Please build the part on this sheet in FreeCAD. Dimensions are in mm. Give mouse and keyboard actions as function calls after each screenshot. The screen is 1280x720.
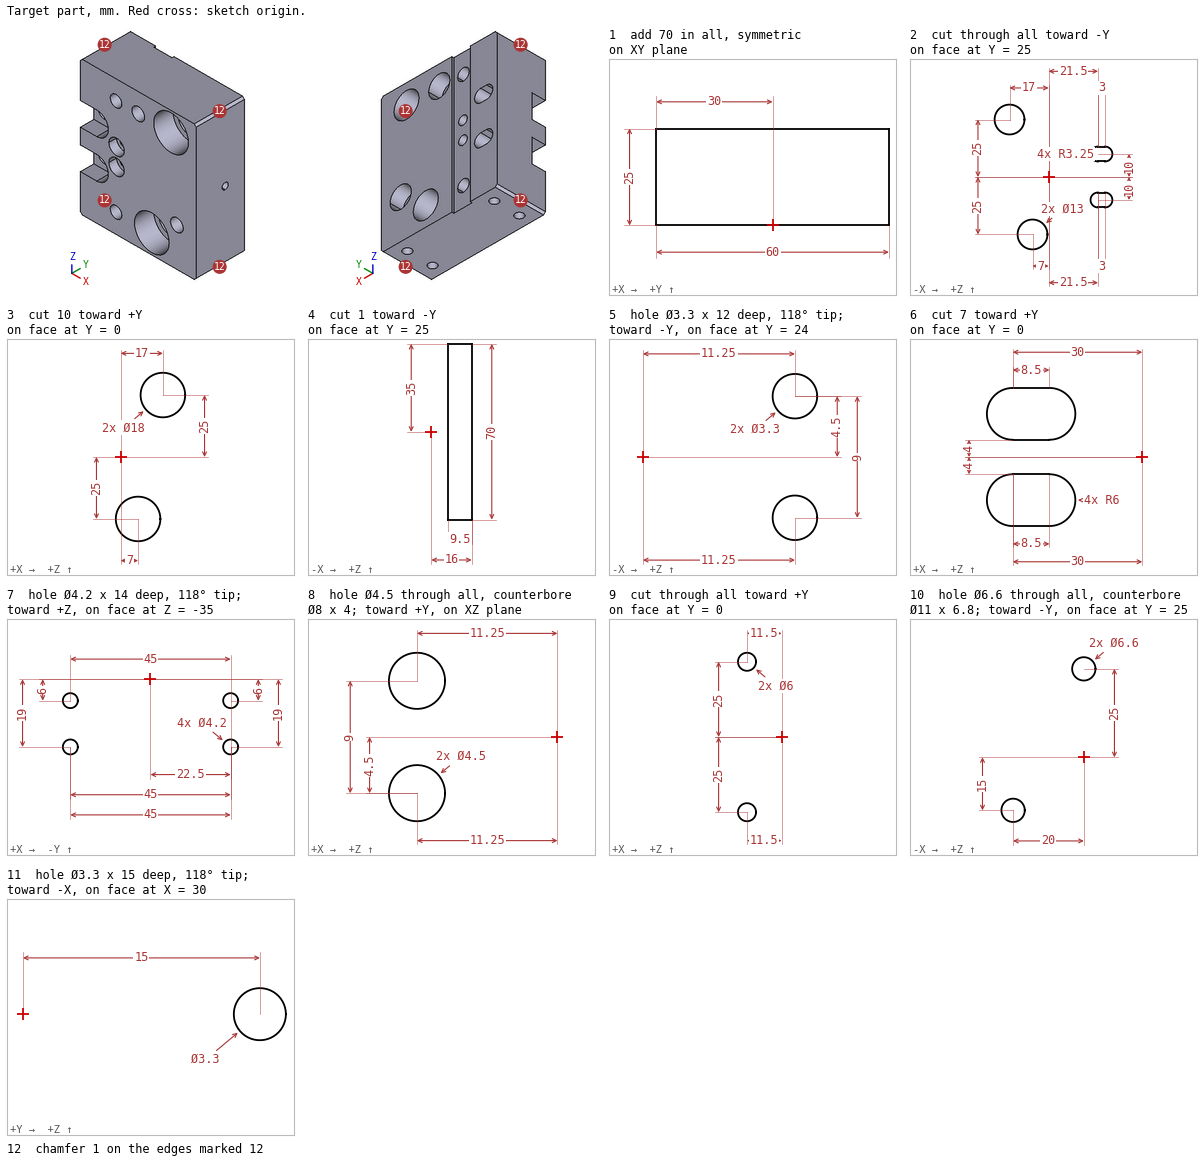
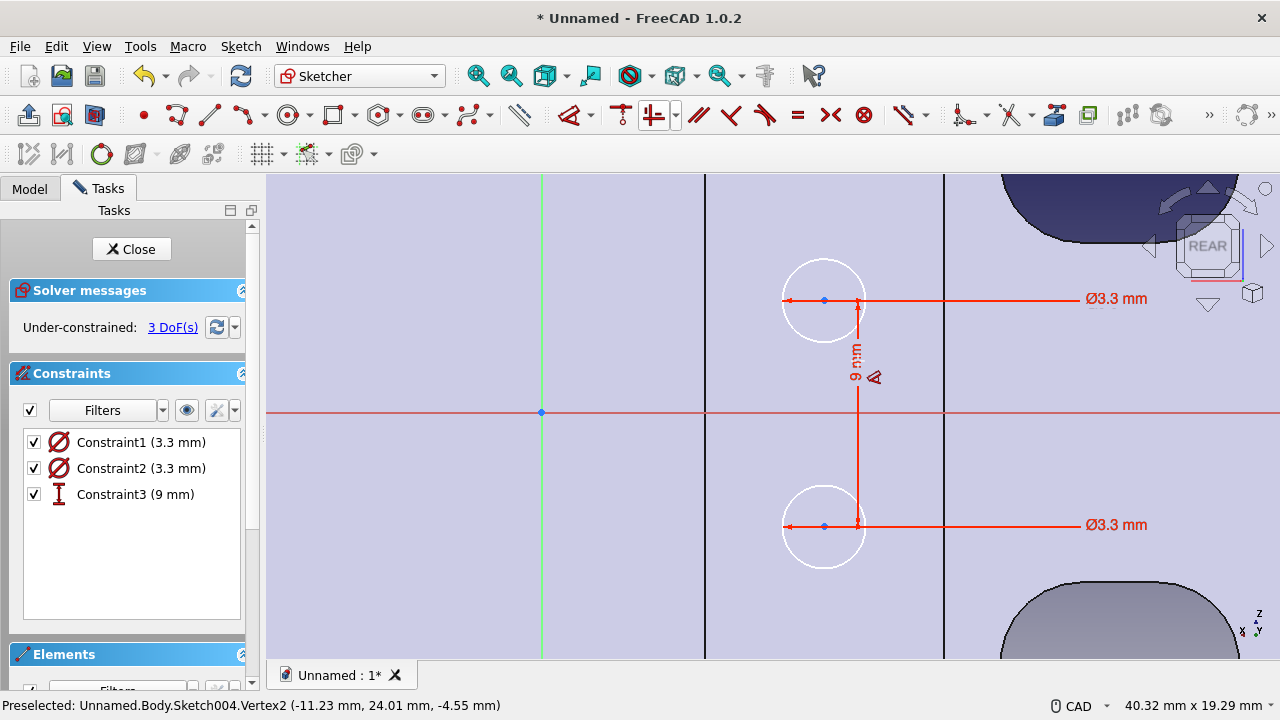
click(824, 301)
click(508, 357)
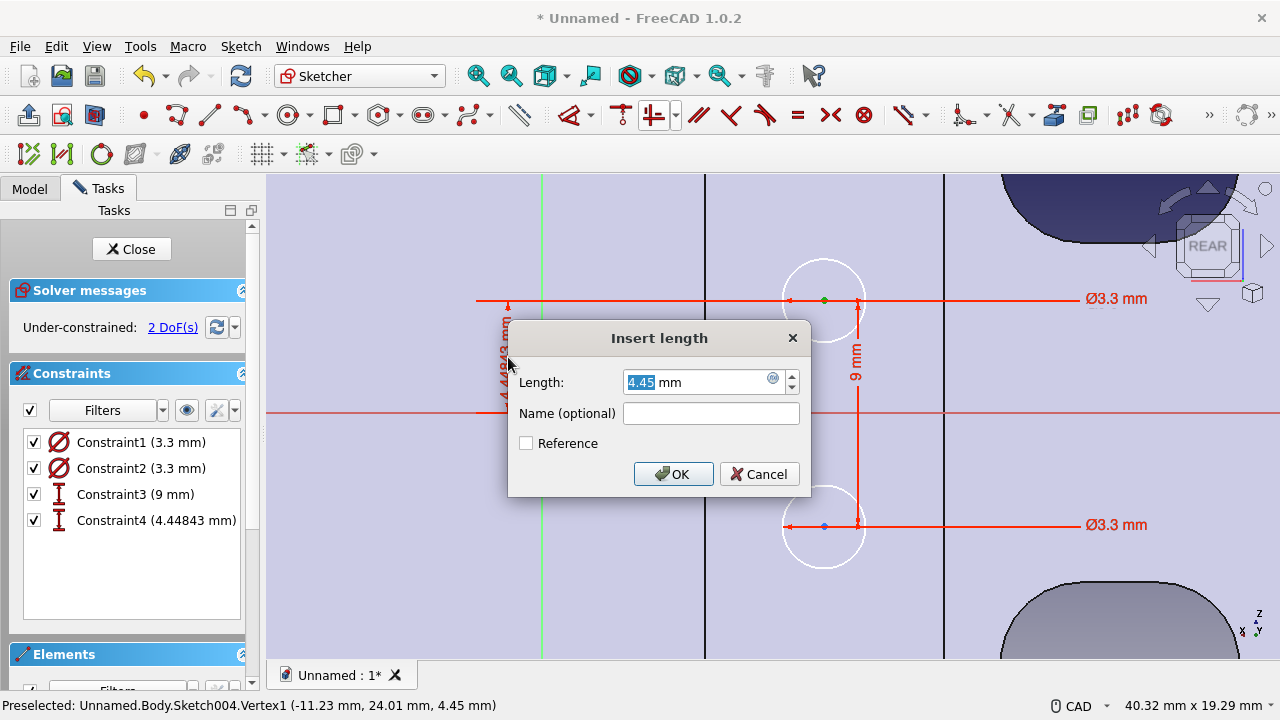
text(4.5)
key(Return)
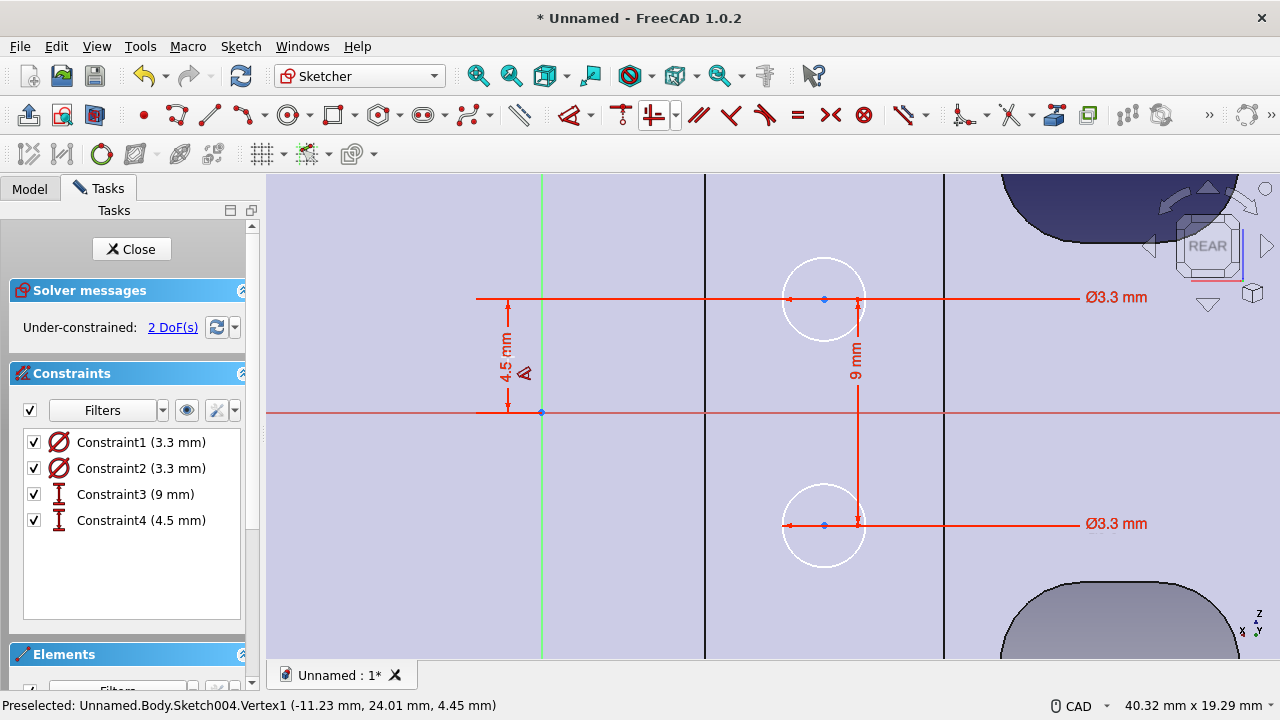
click(824, 299)
click(683, 265)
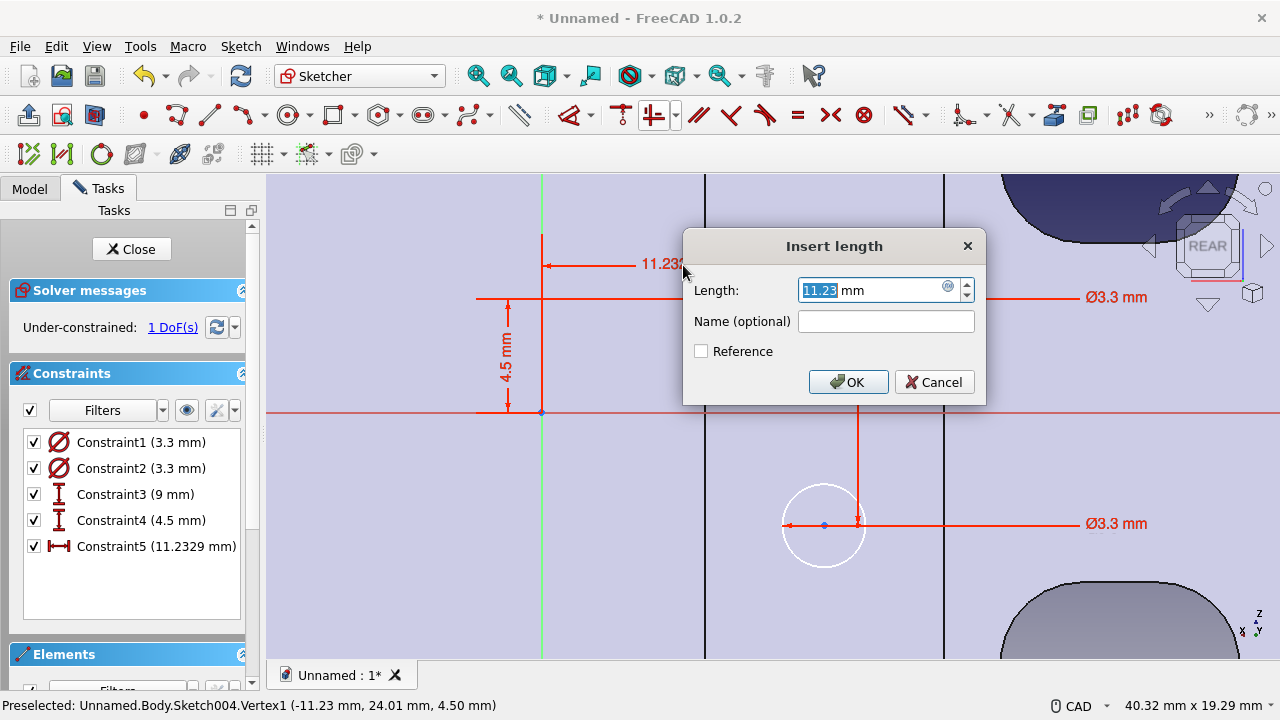
text(11.25)
key(Return)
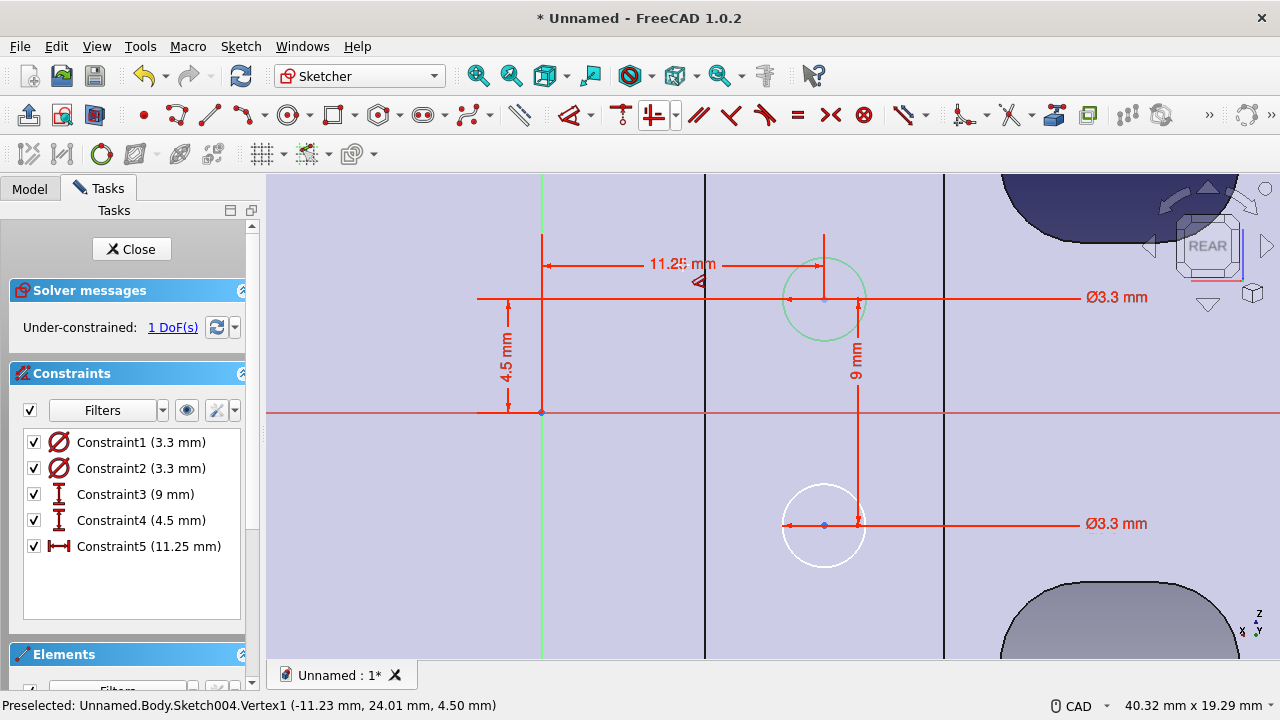
click(824, 526)
click(683, 560)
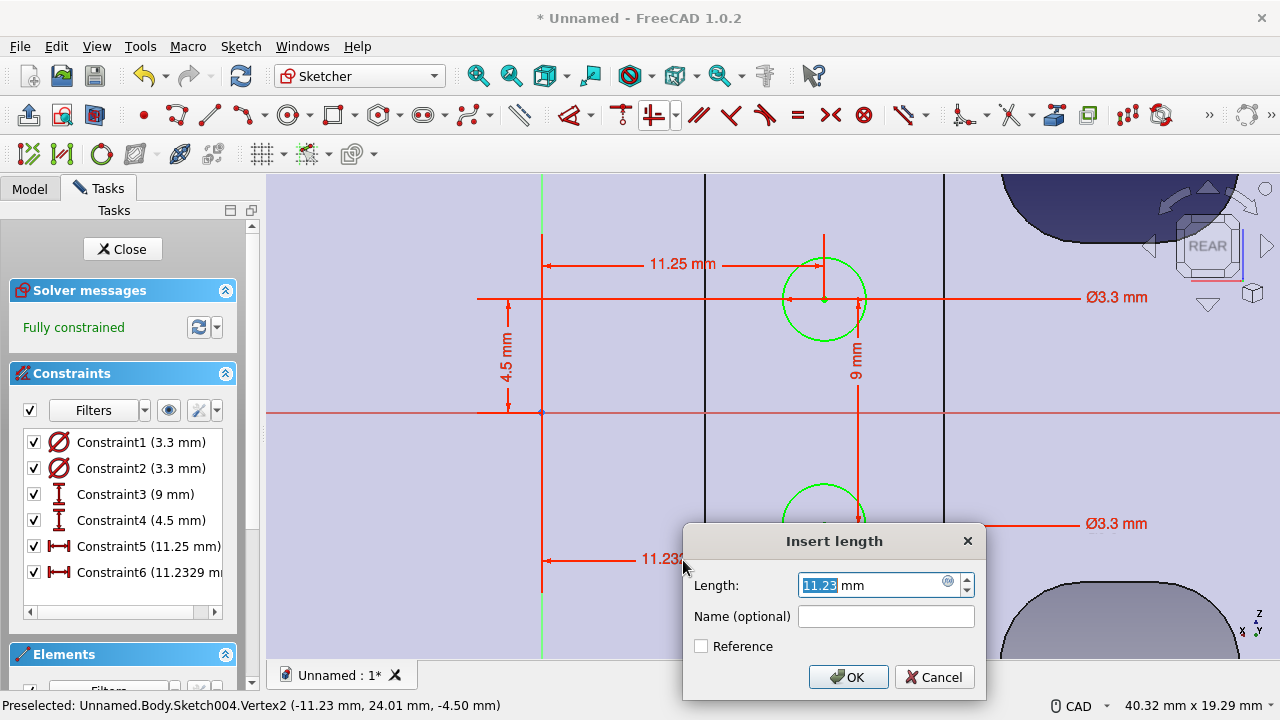
text(11.25)
key(Return)
key(Escape)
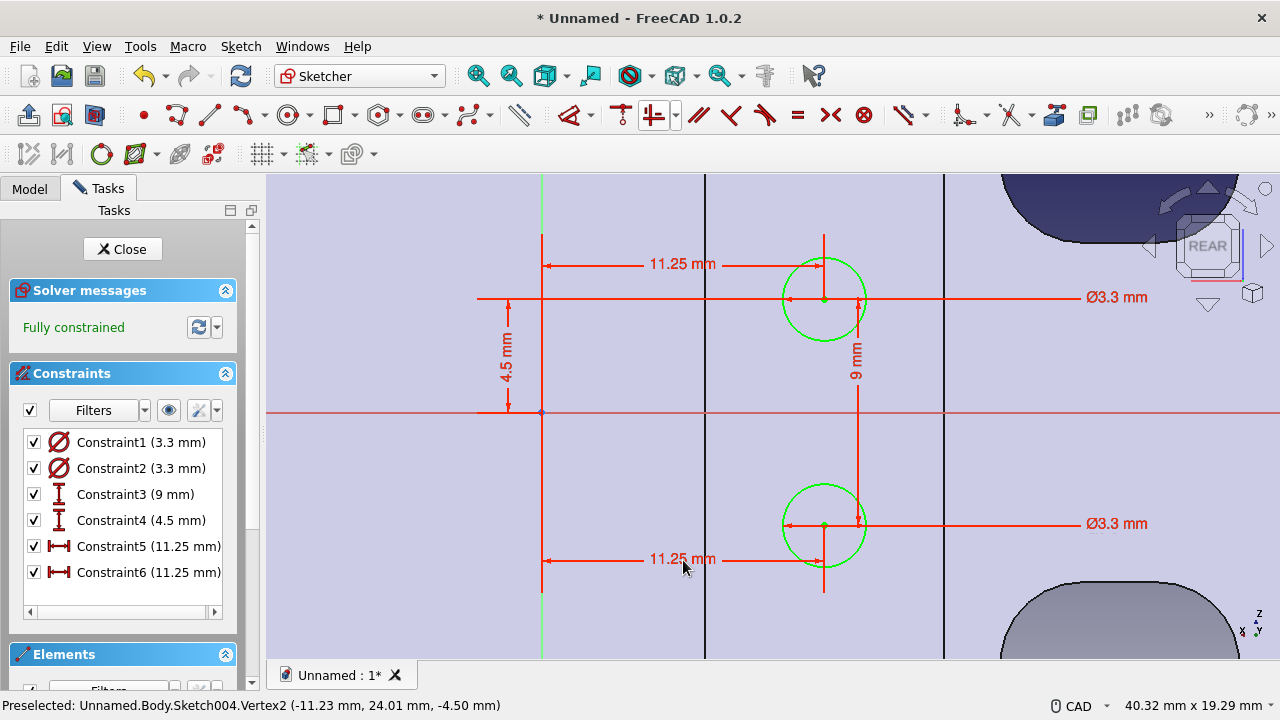
click(123, 249)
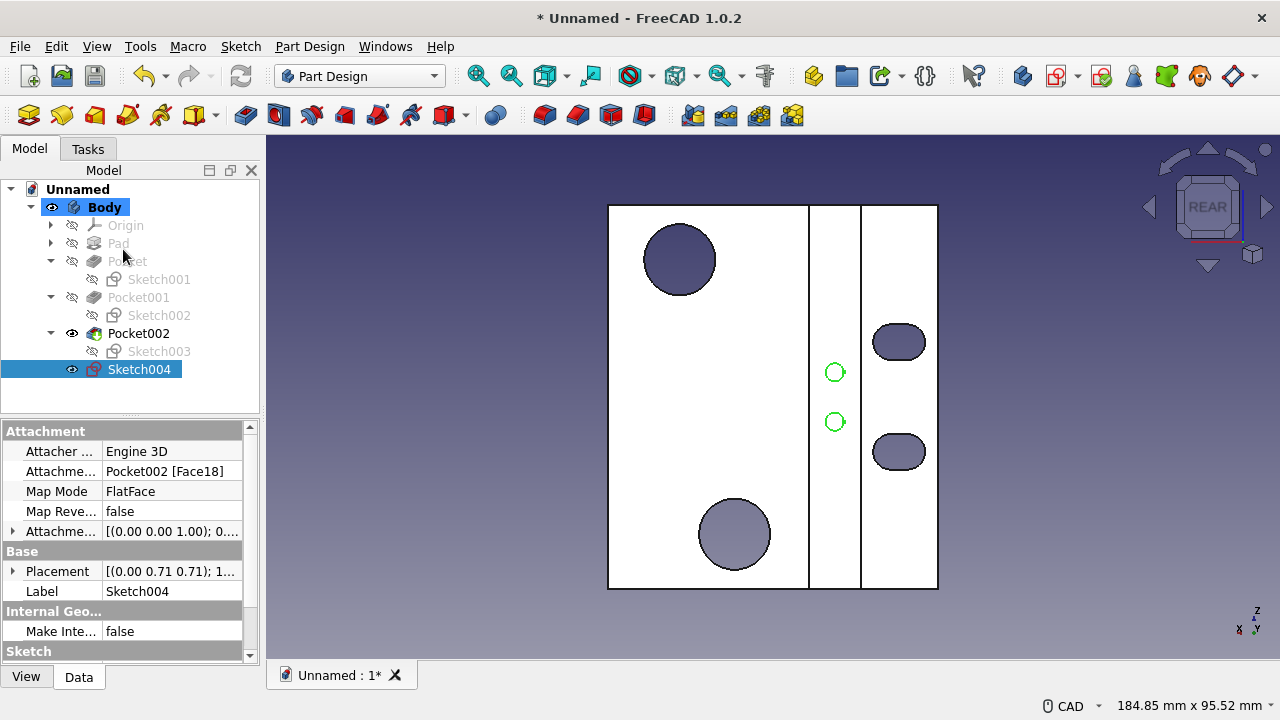
click(279, 116)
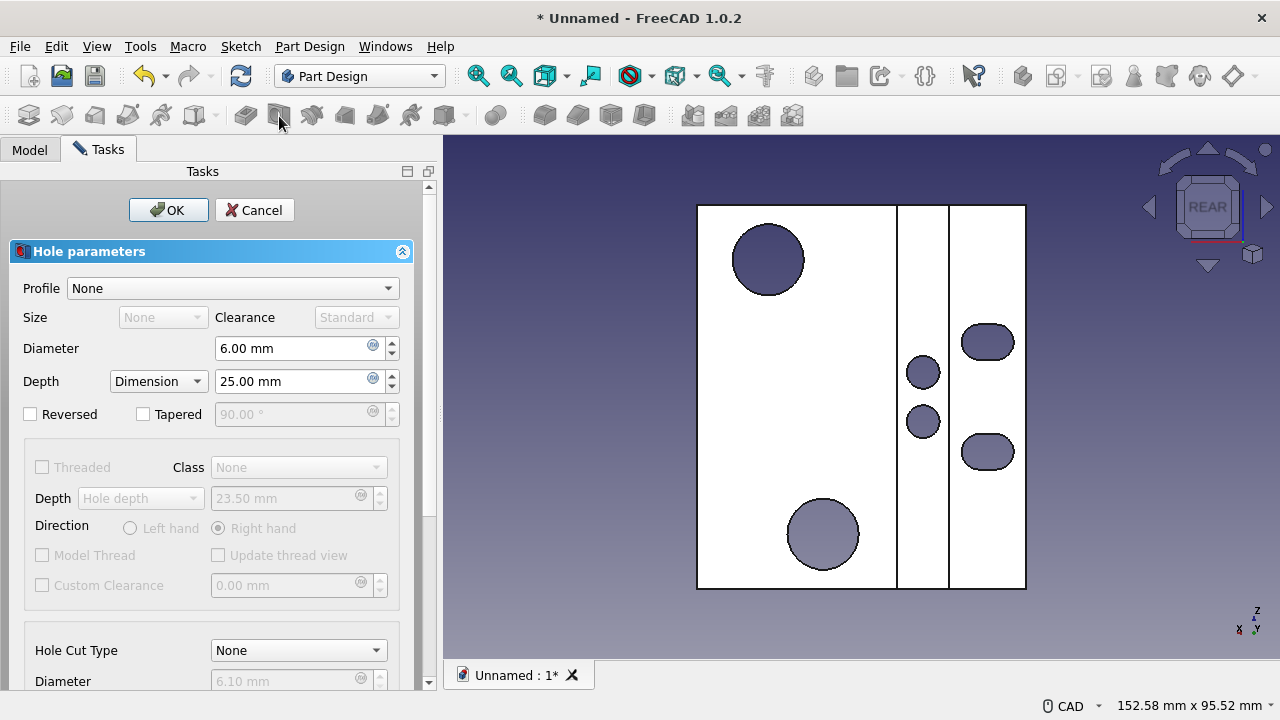
triple_click(300, 348)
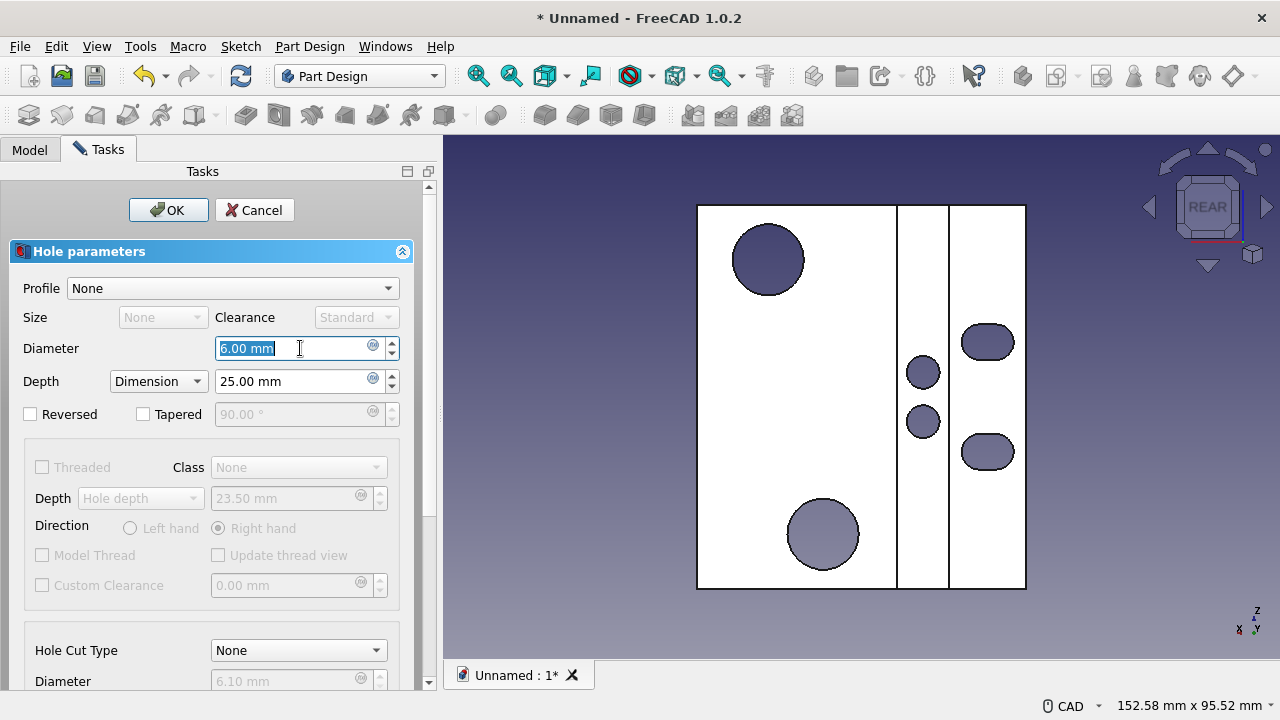
text(3.3)
key(Tab)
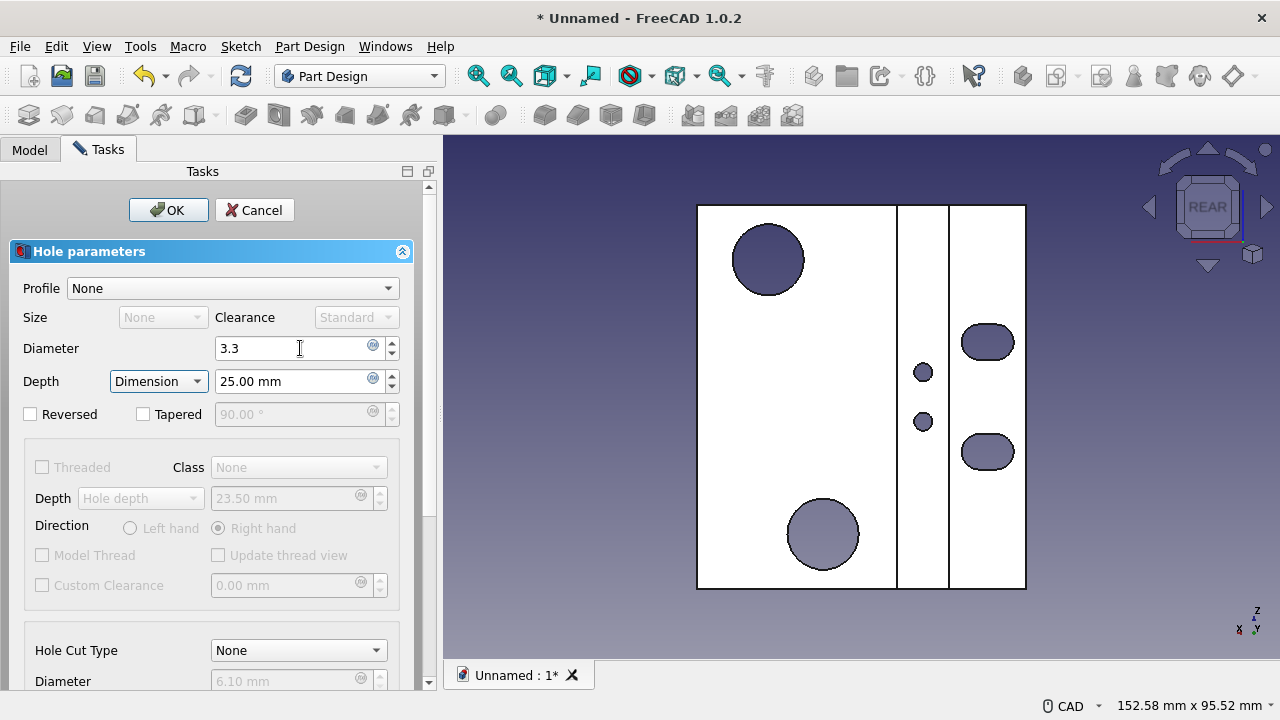
triple_click(300, 382)